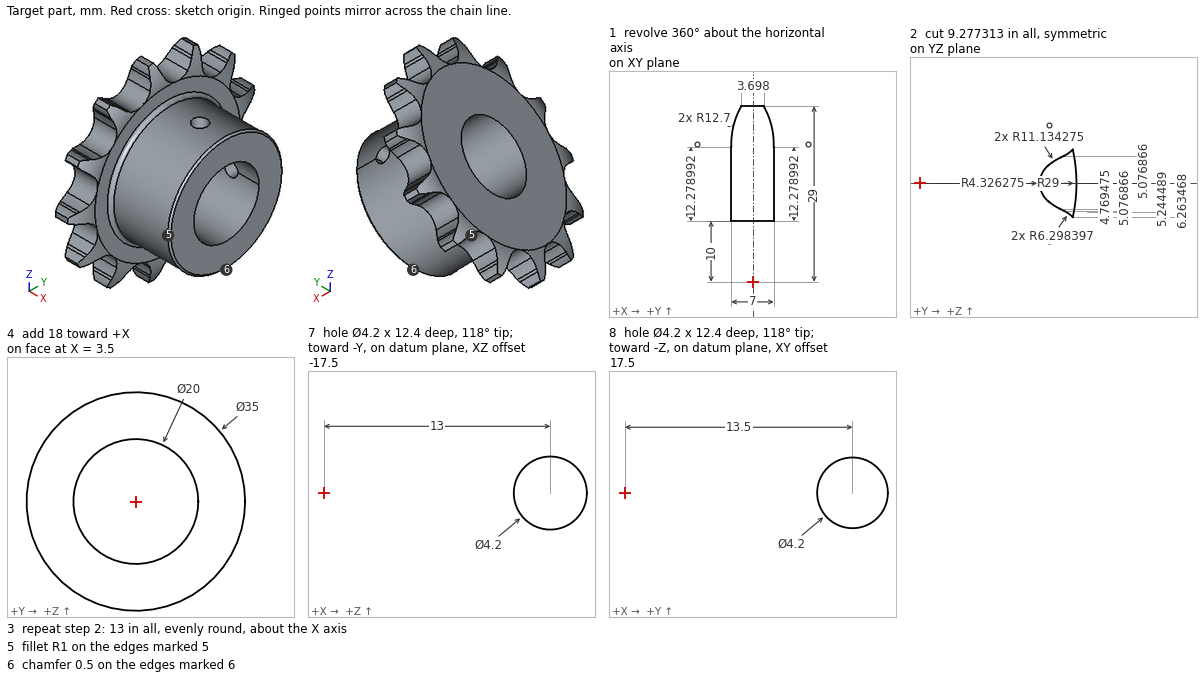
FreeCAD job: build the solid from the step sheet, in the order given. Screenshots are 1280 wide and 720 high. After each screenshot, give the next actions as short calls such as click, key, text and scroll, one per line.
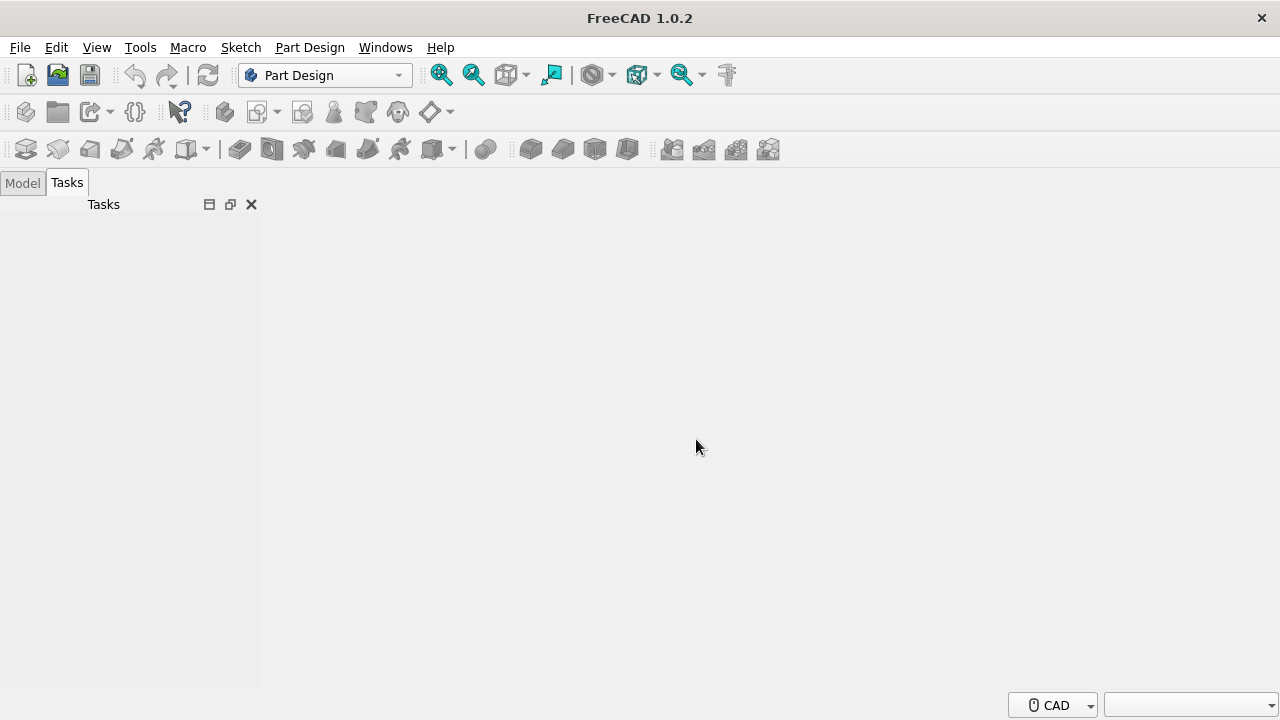
key(ctrl+n)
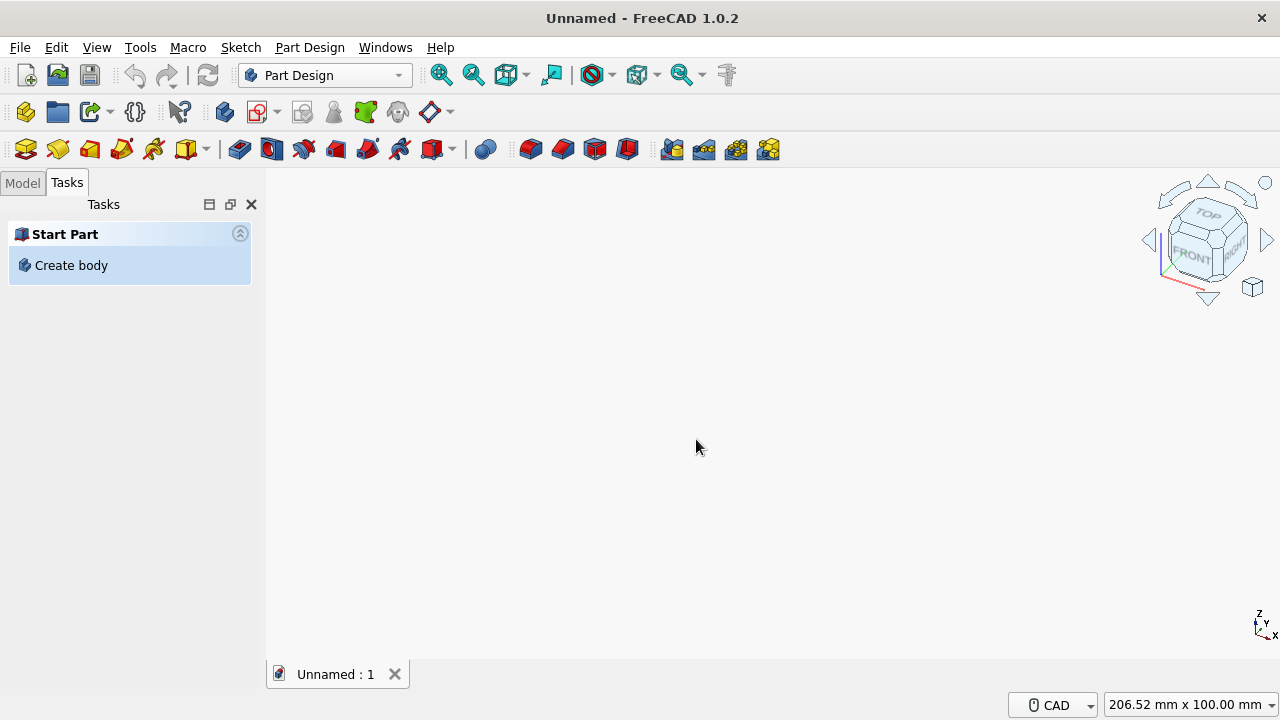
click(258, 112)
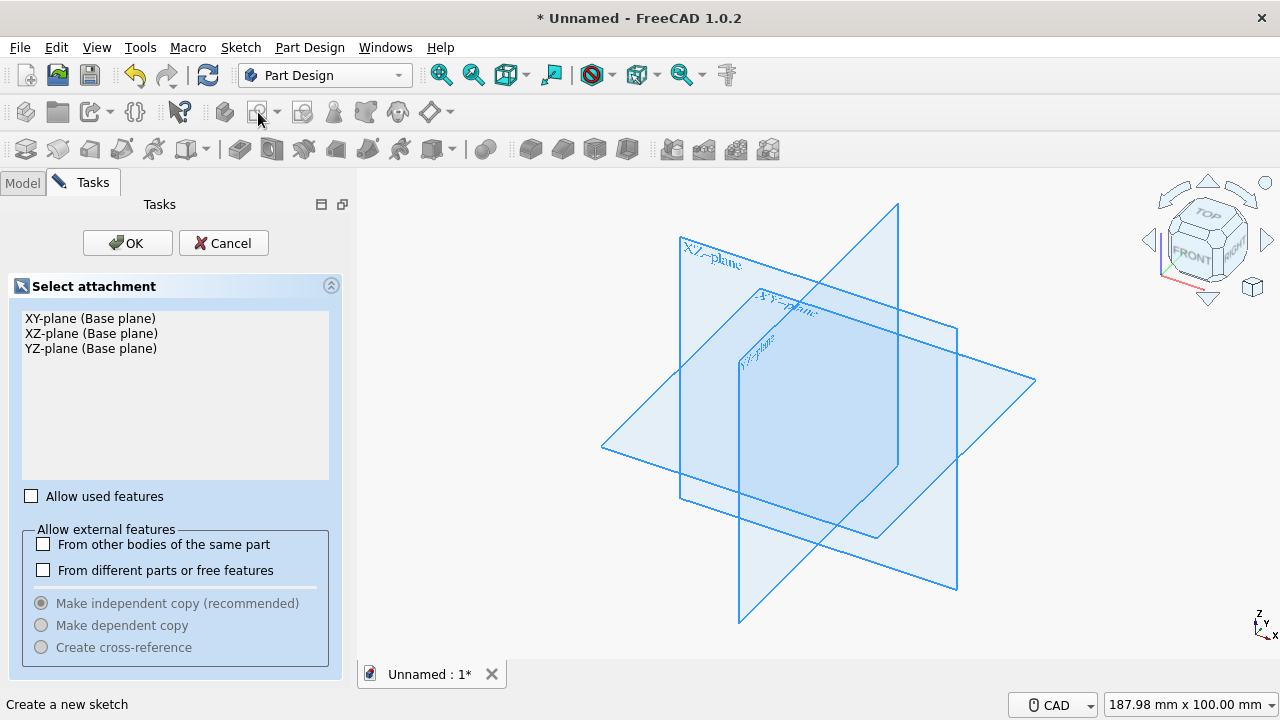
click(82, 318)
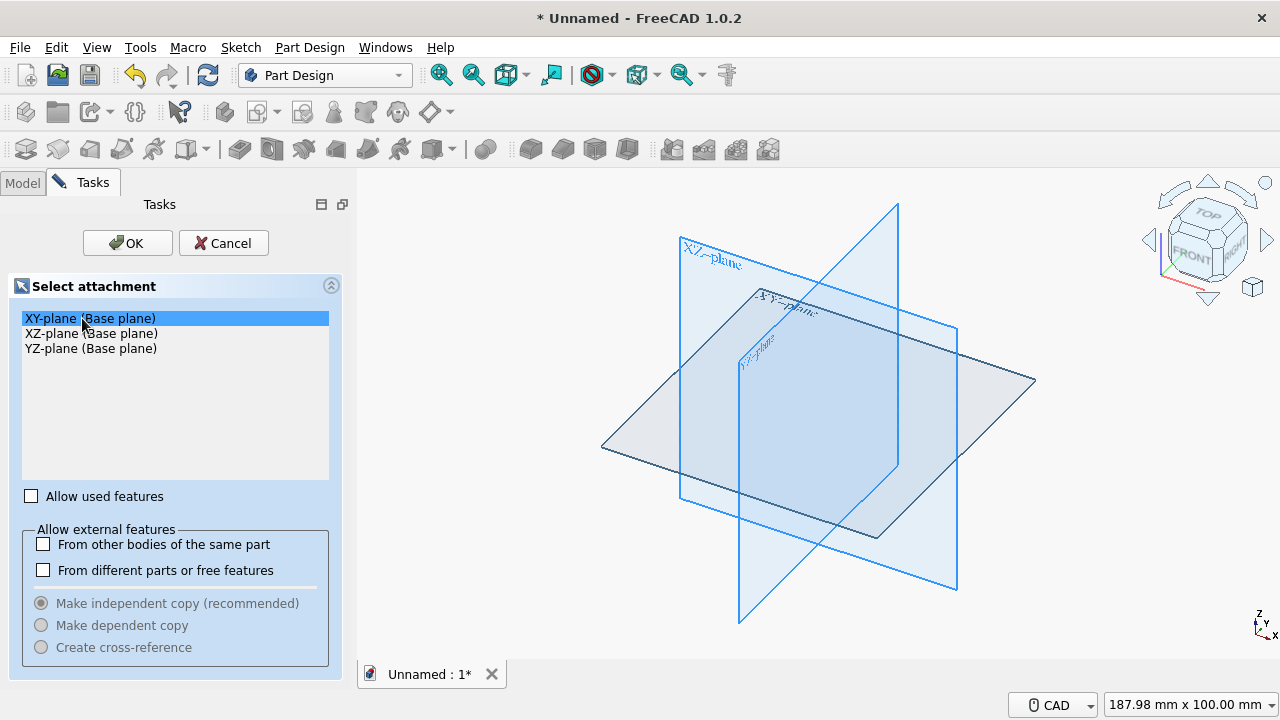
click(128, 243)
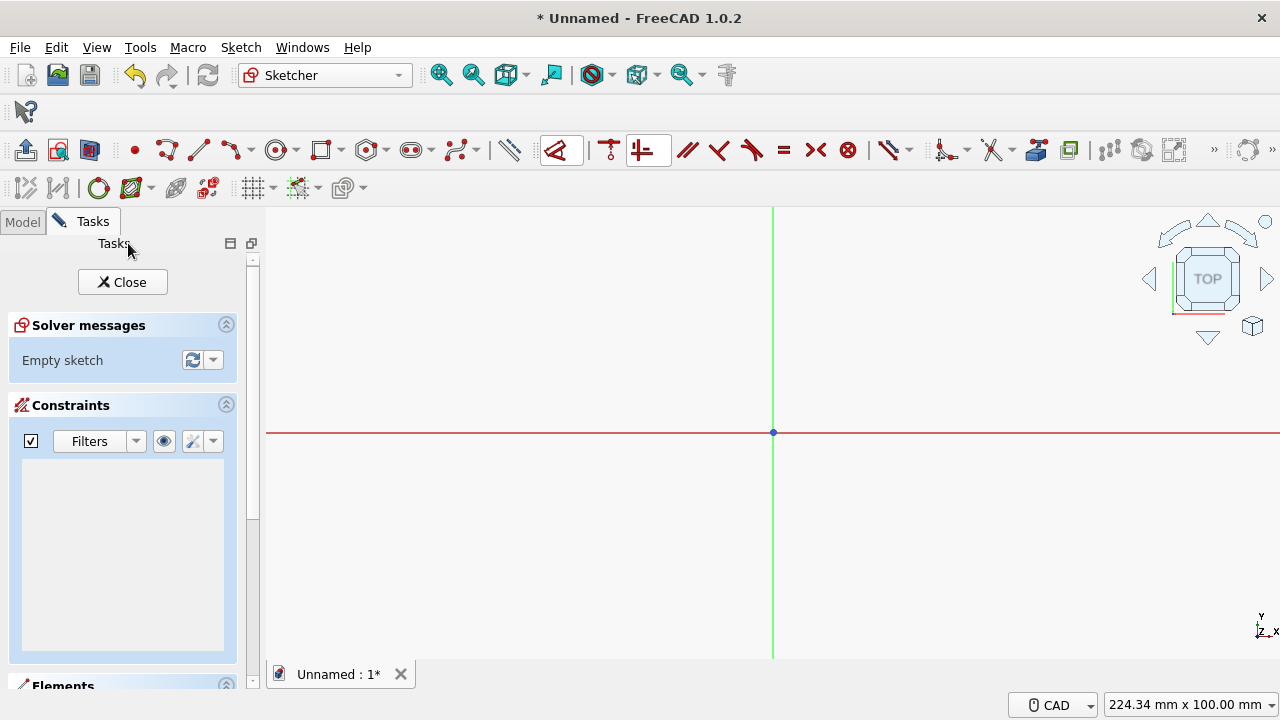
scroll(829, 314, up, 4)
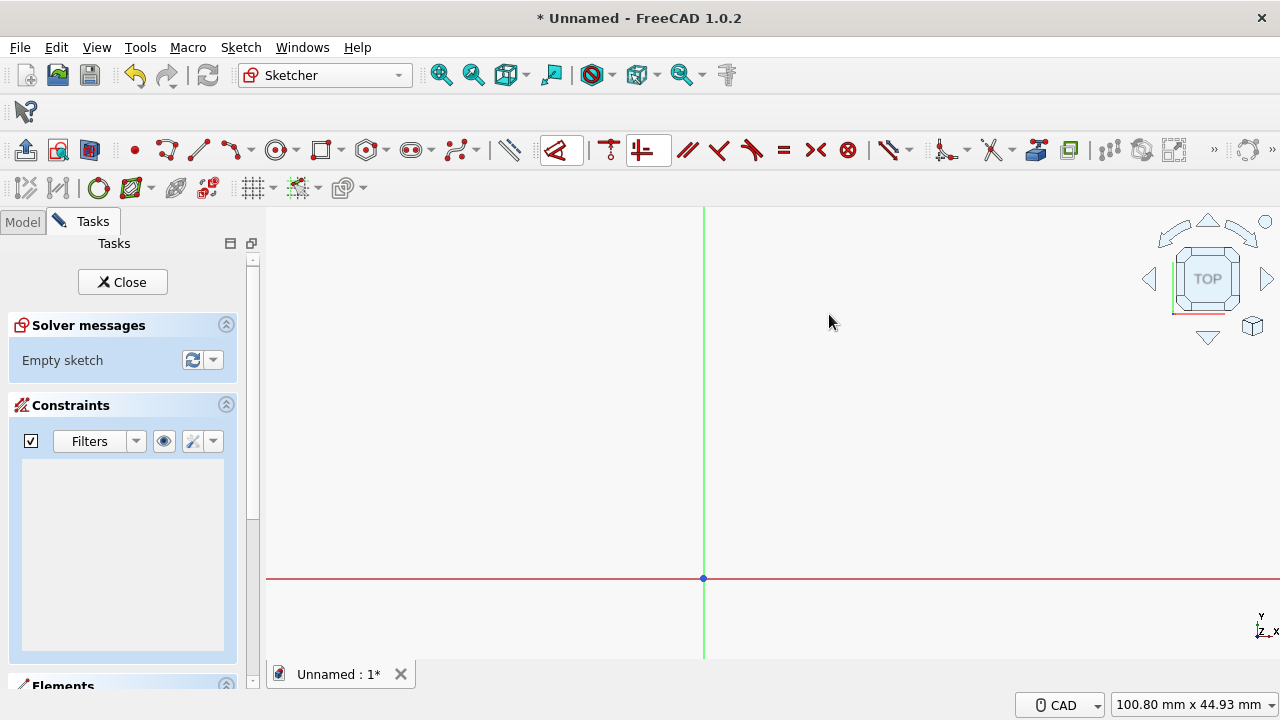
click(168, 150)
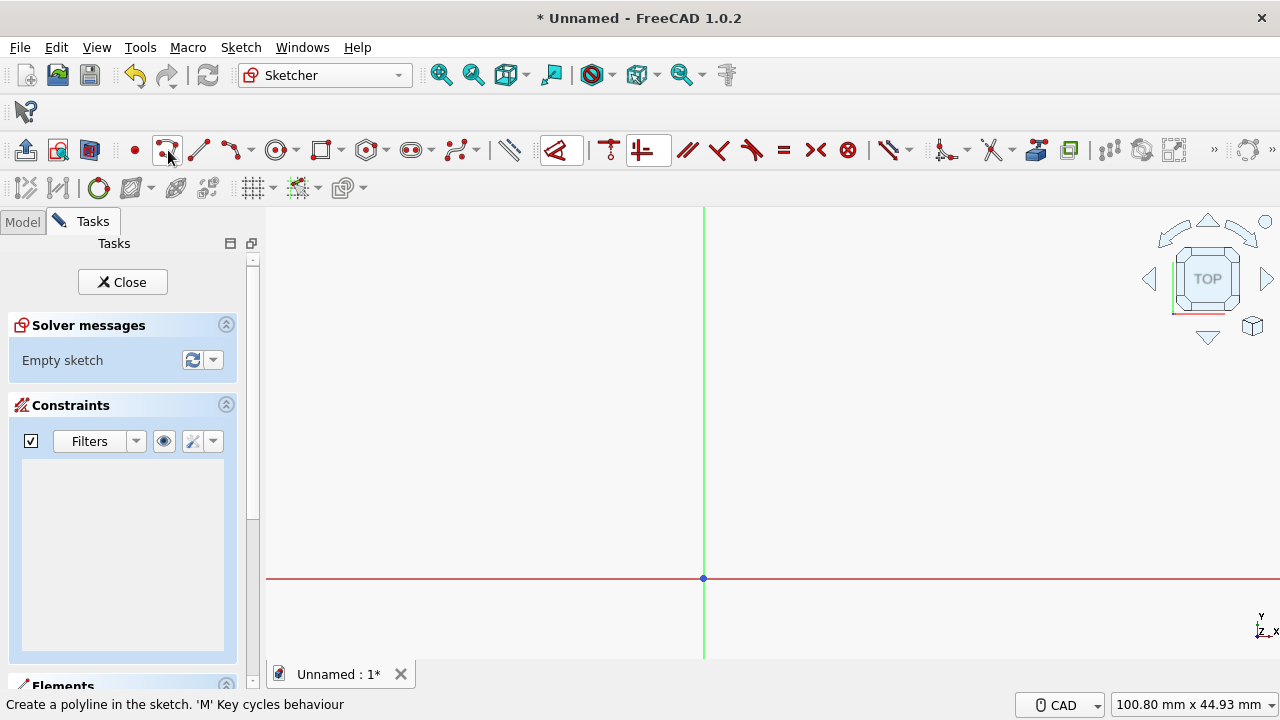
click(668, 354)
click(668, 478)
click(739, 478)
click(739, 354)
right_click(739, 354)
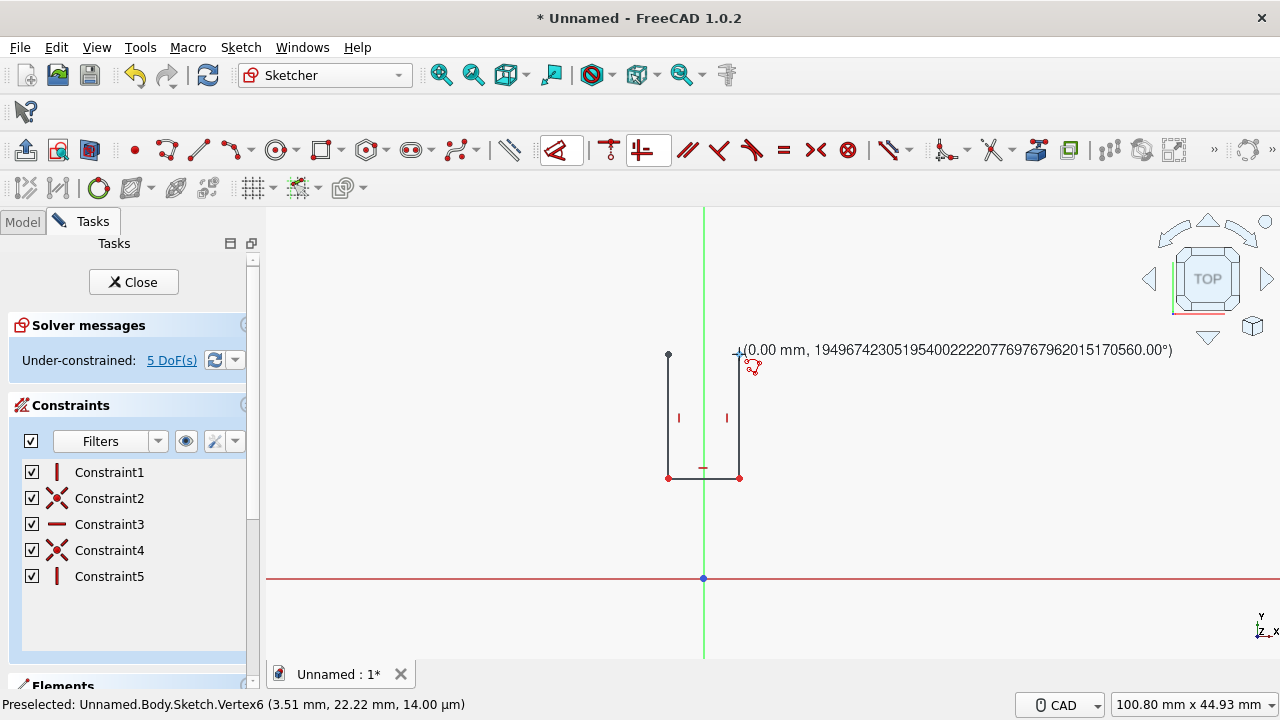
click(200, 150)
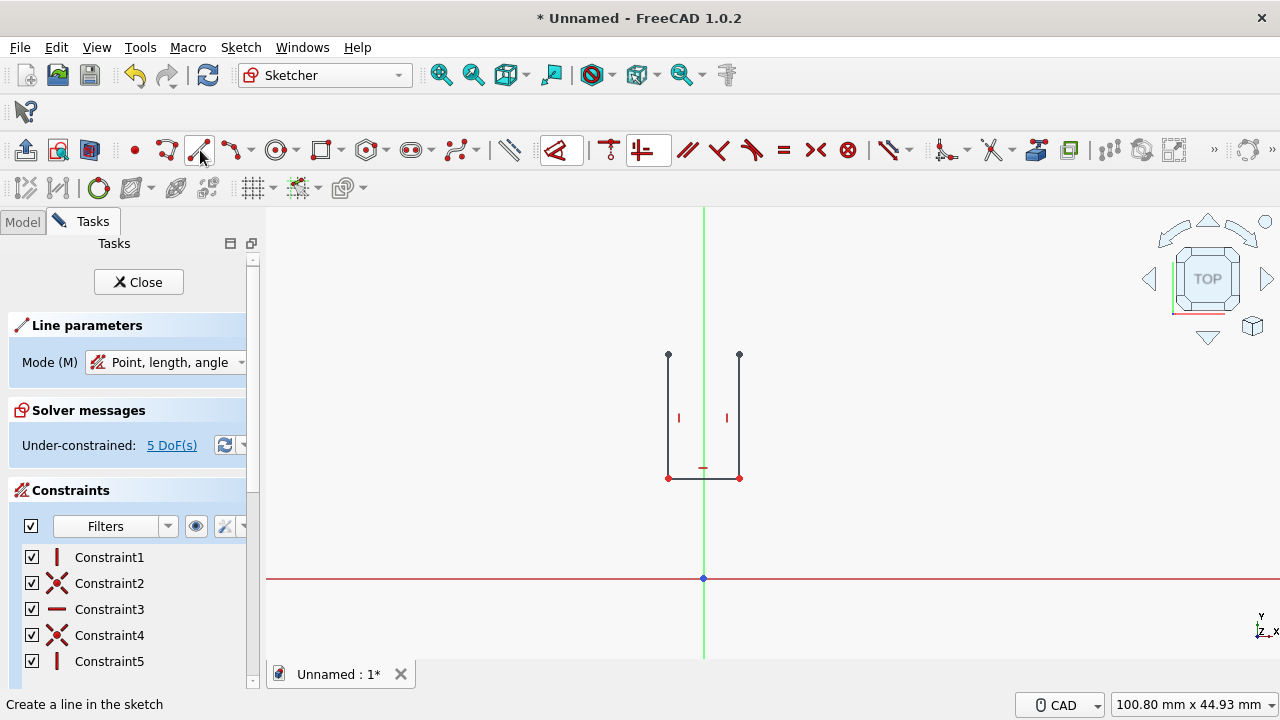
click(722, 287)
click(685, 287)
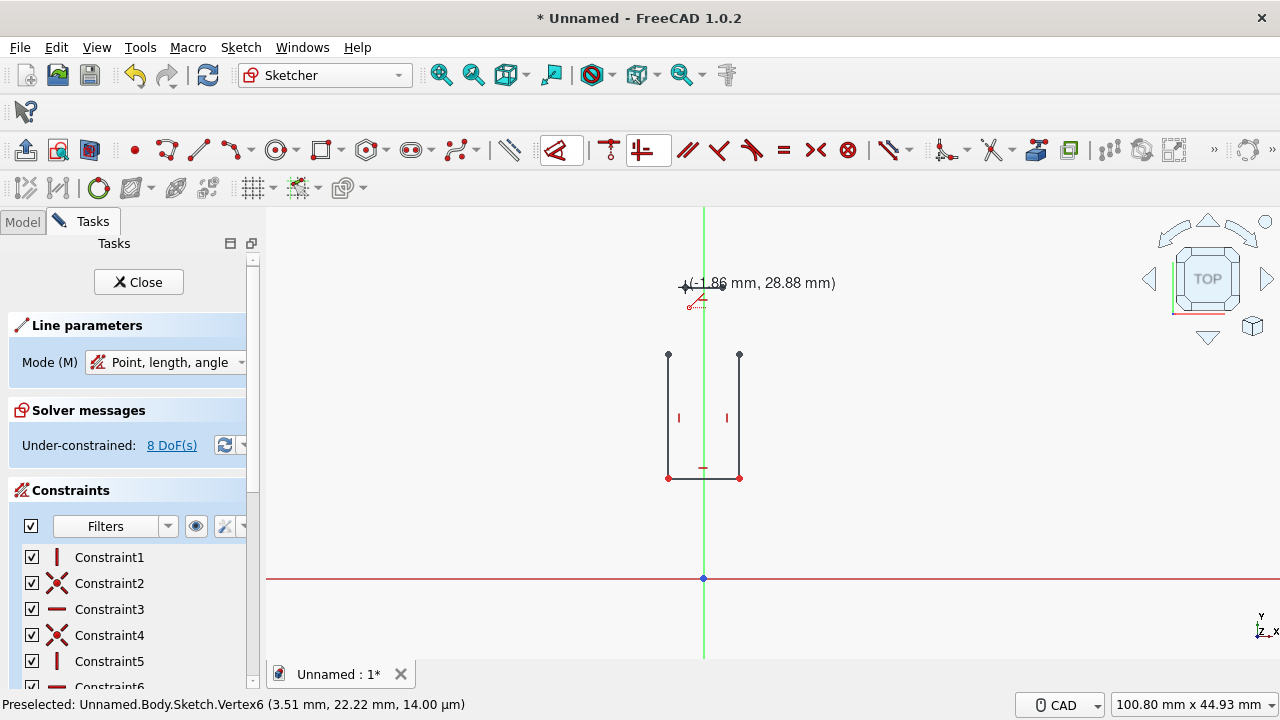
click(232, 150)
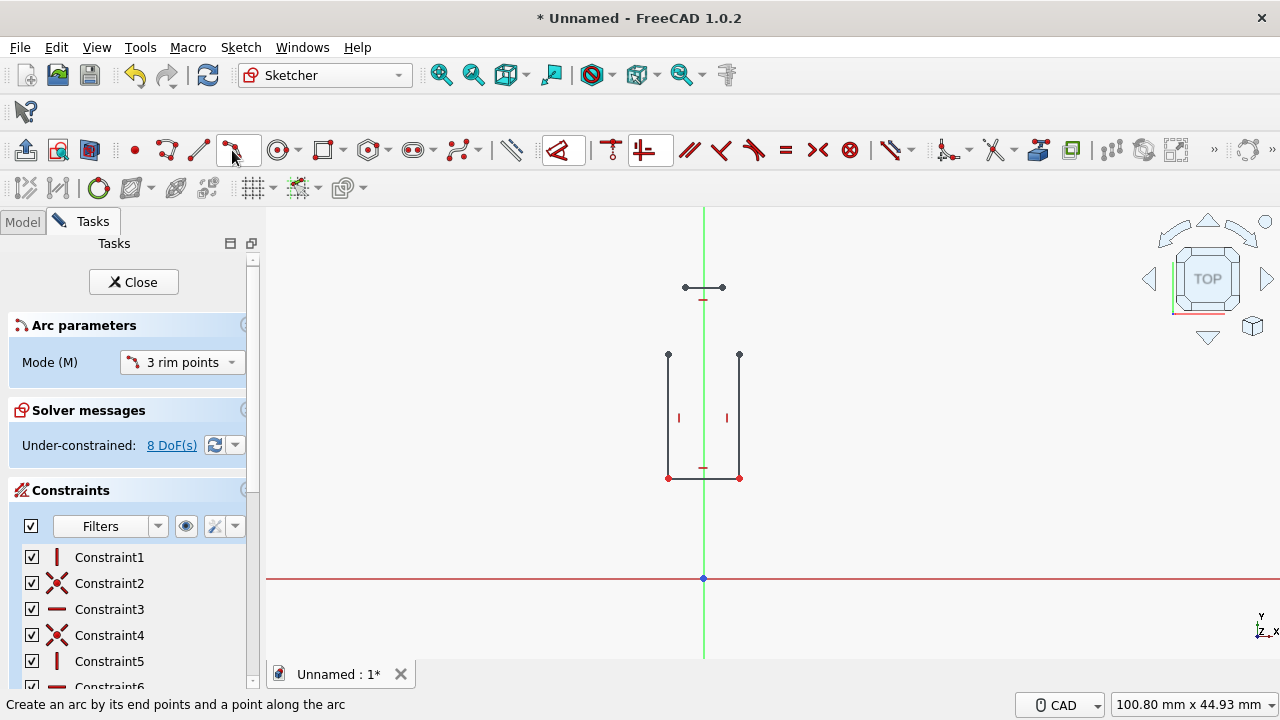
click(739, 355)
click(722, 288)